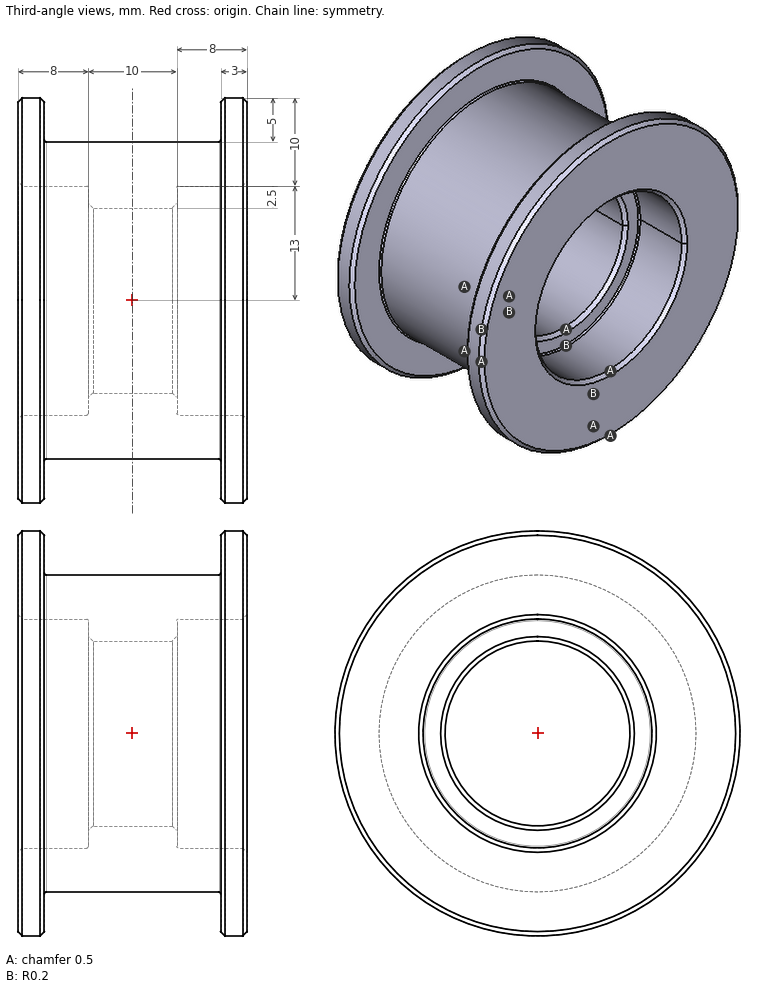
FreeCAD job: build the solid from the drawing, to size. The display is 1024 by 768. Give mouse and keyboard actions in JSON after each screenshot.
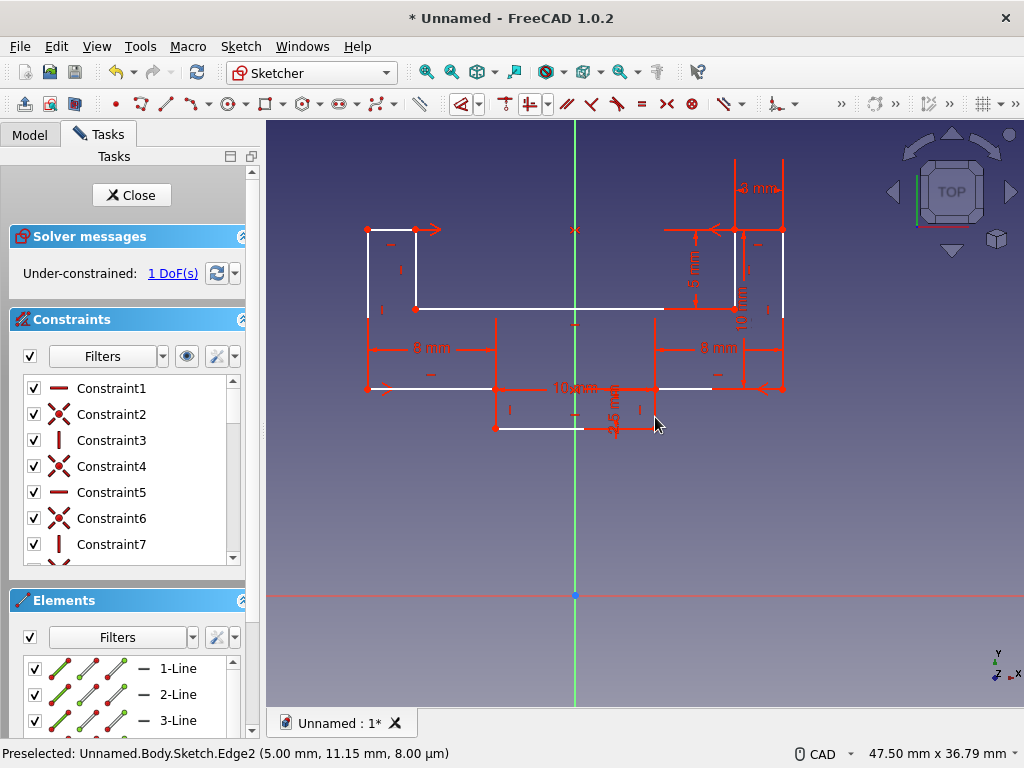
{"action": "left_click", "coordinate": [655, 389]}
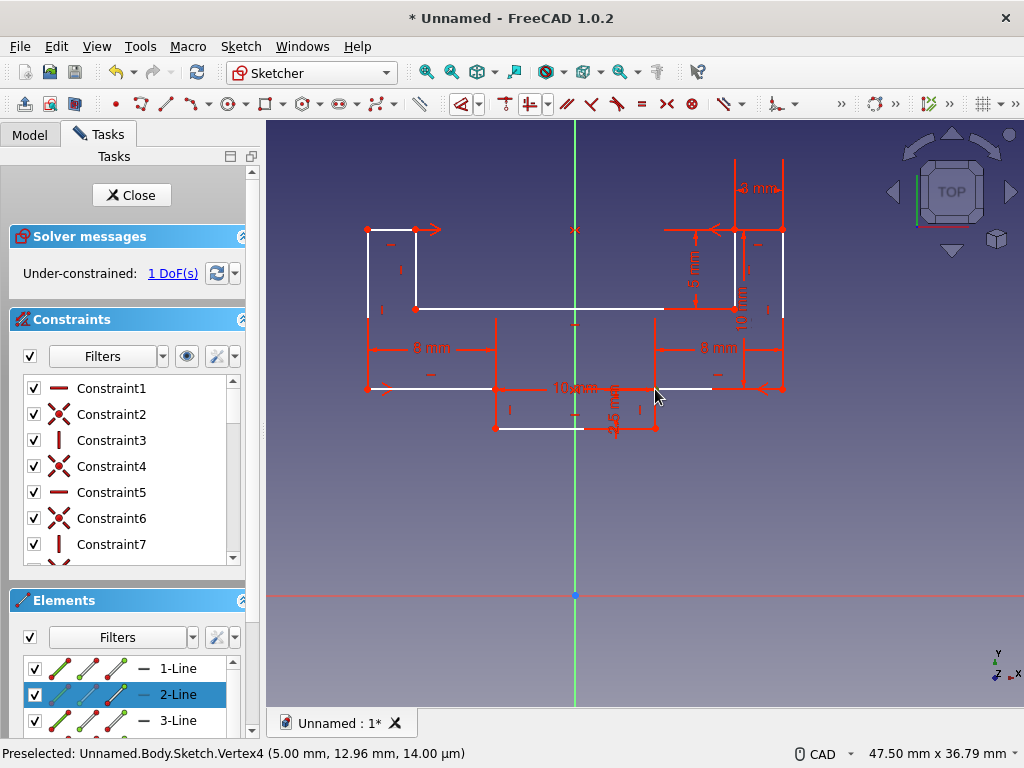
{"action": "key", "text": "i"}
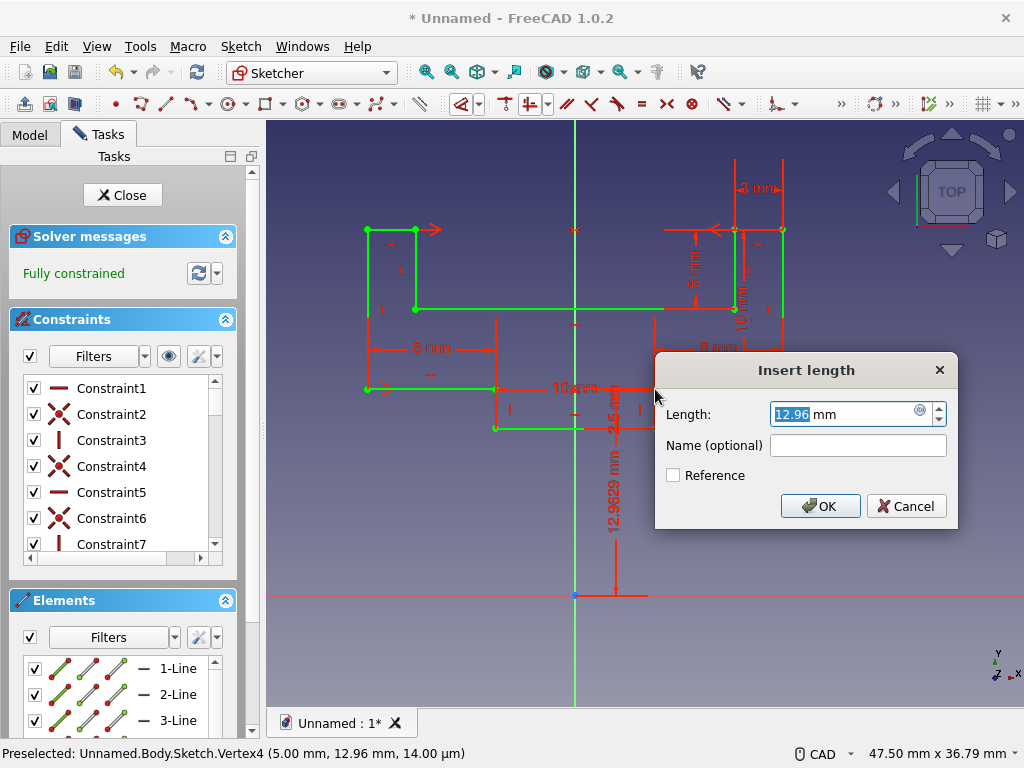
{"action": "type", "text": "13"}
{"action": "key", "text": "Return"}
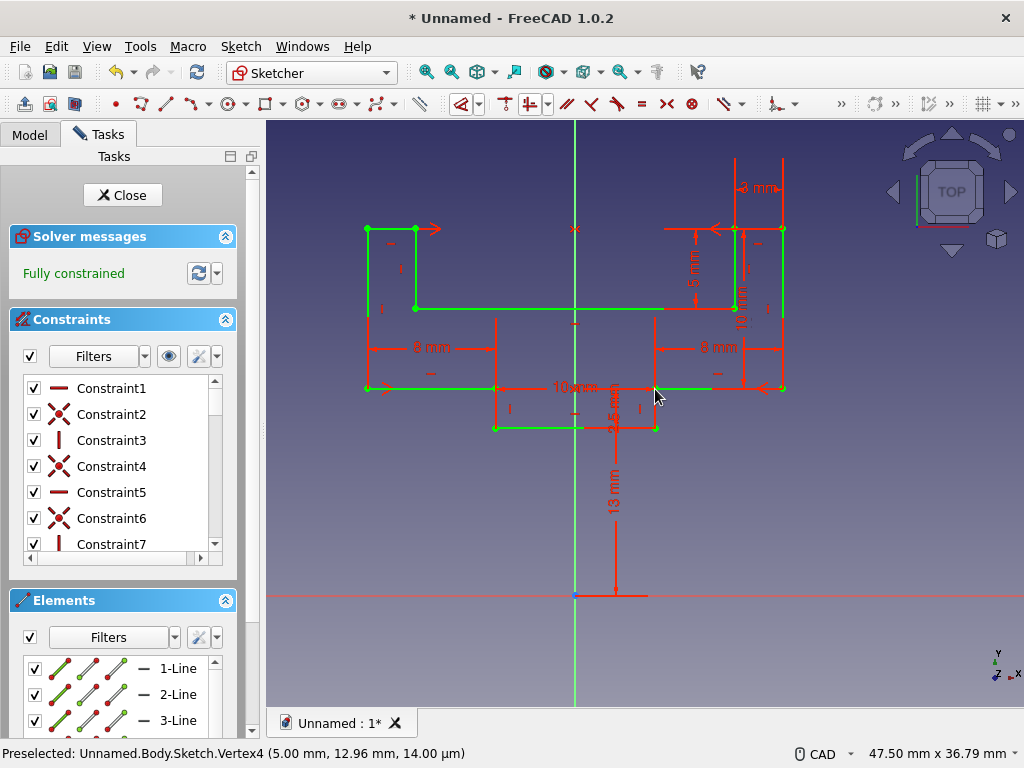
{"action": "left_click", "coordinate": [123, 195]}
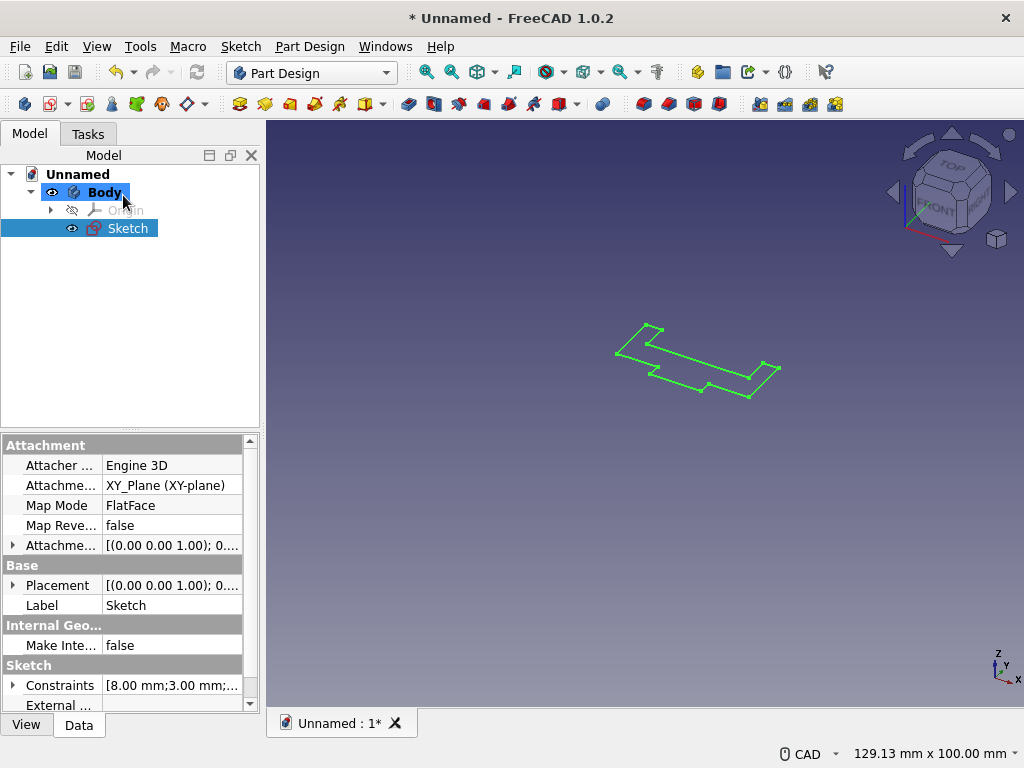
{"action": "left_click", "coordinate": [265, 104]}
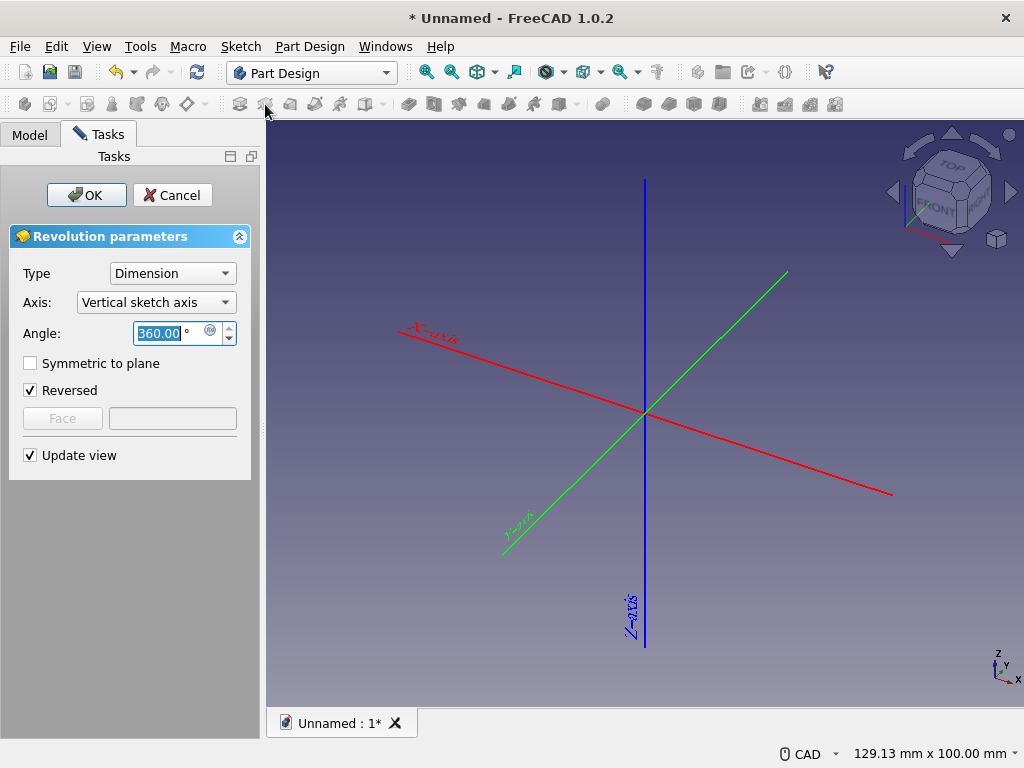
{"action": "left_click", "coordinate": [157, 302]}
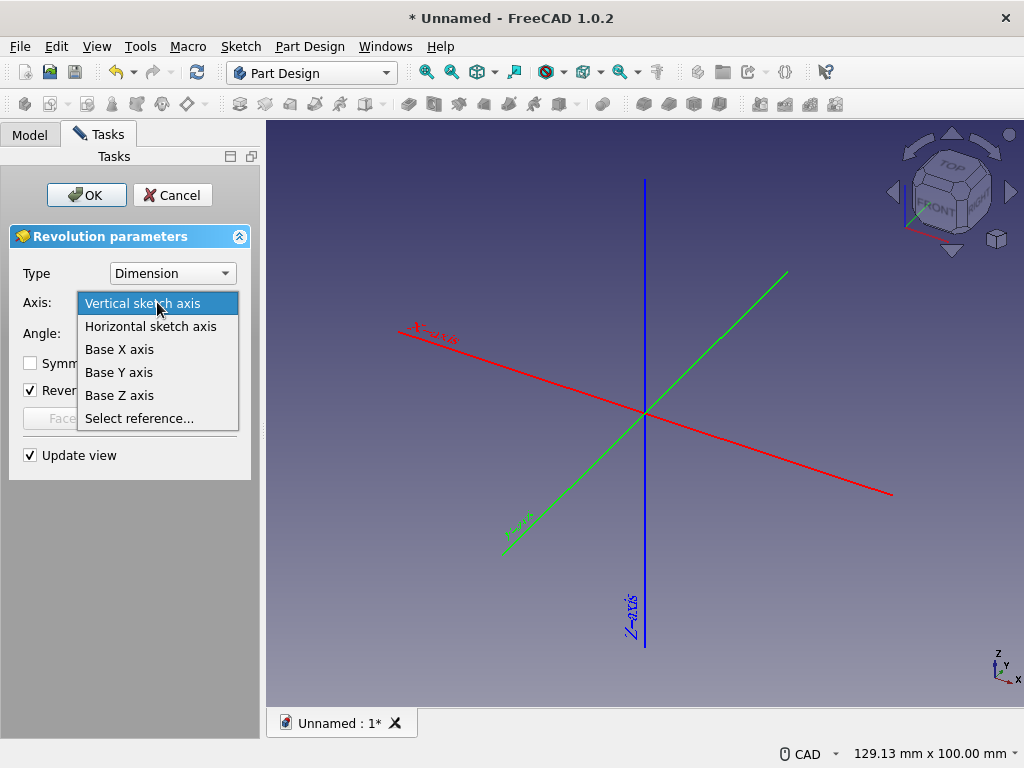
{"action": "left_click", "coordinate": [156, 326]}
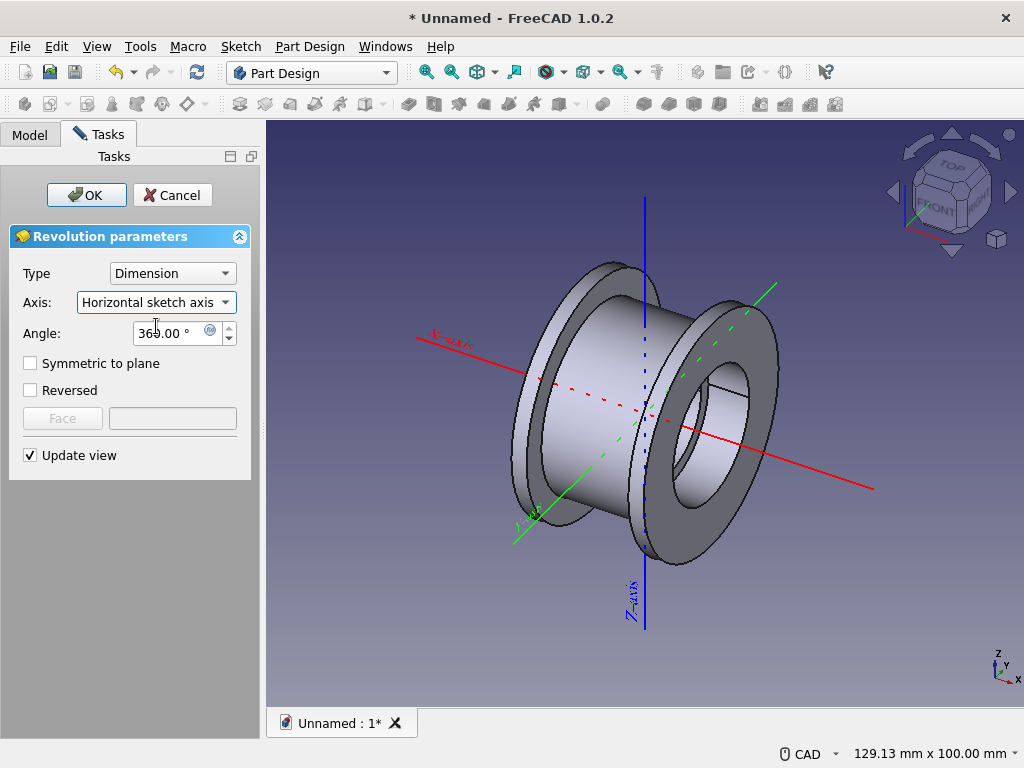
{"action": "left_click", "coordinate": [87, 195]}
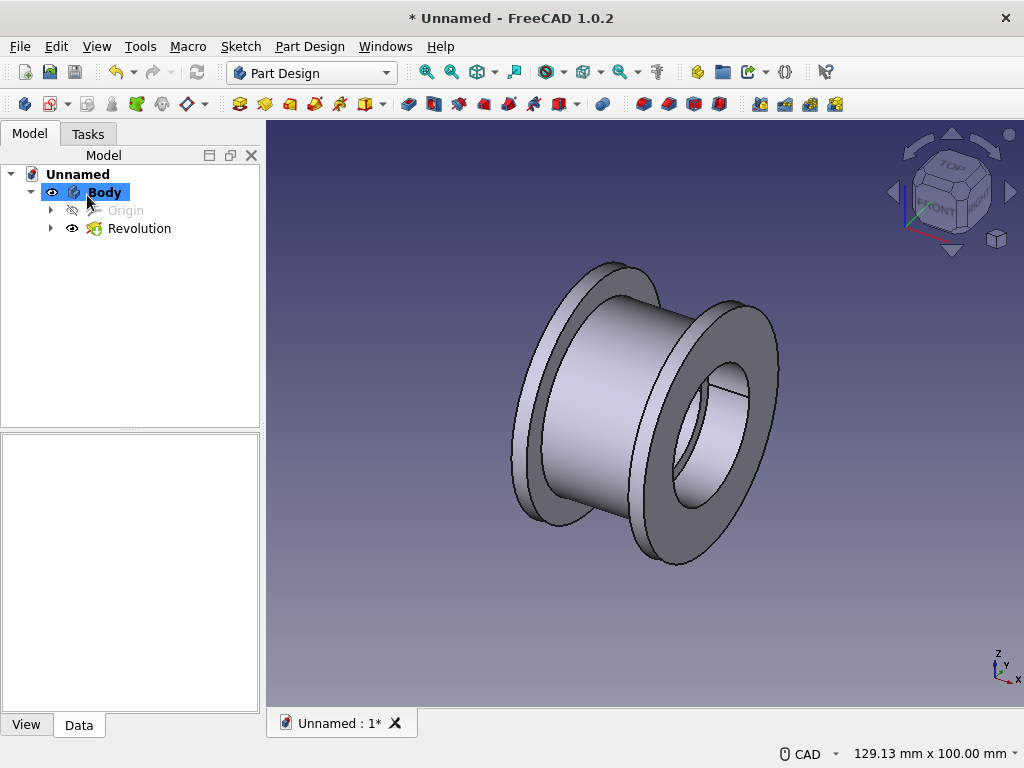
{"action": "left_click", "coordinate": [699, 506]}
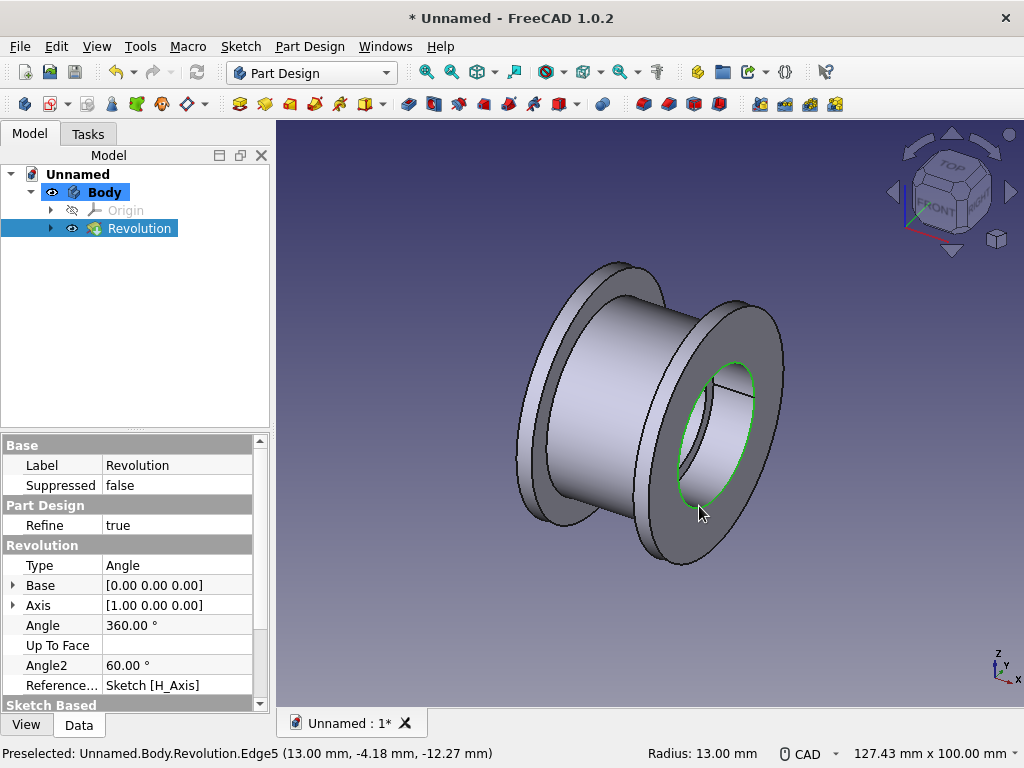
{"action": "left_click", "coordinate": [649, 501], "text": "ctrl"}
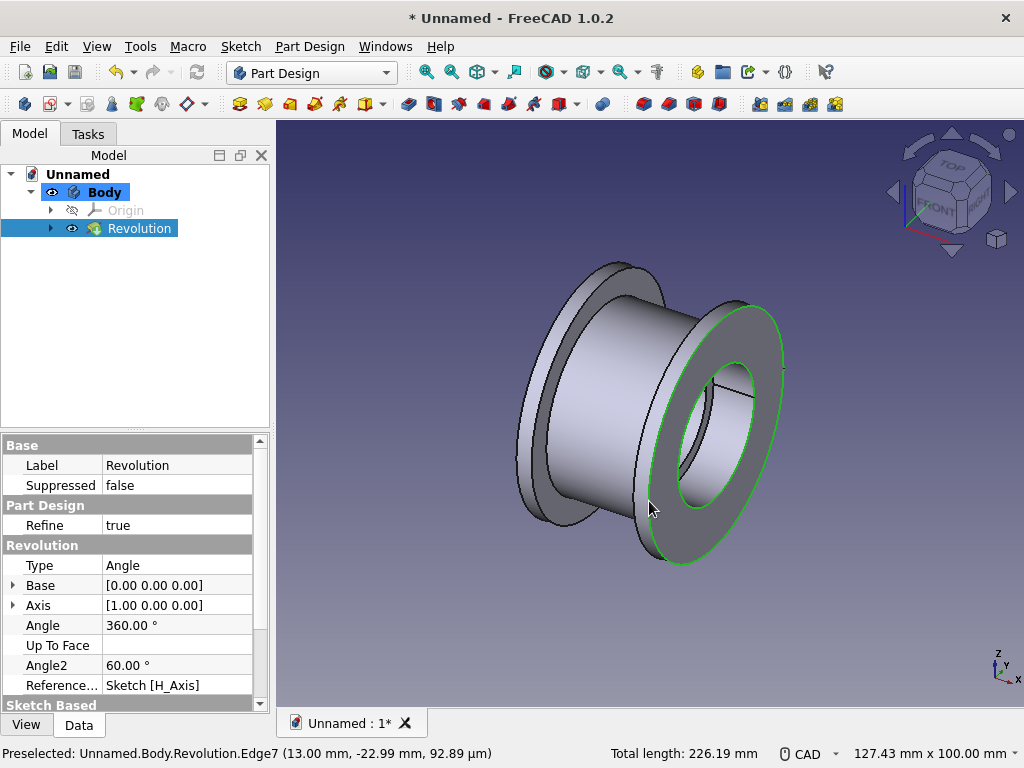
{"action": "left_click", "coordinate": [722, 303], "text": "ctrl"}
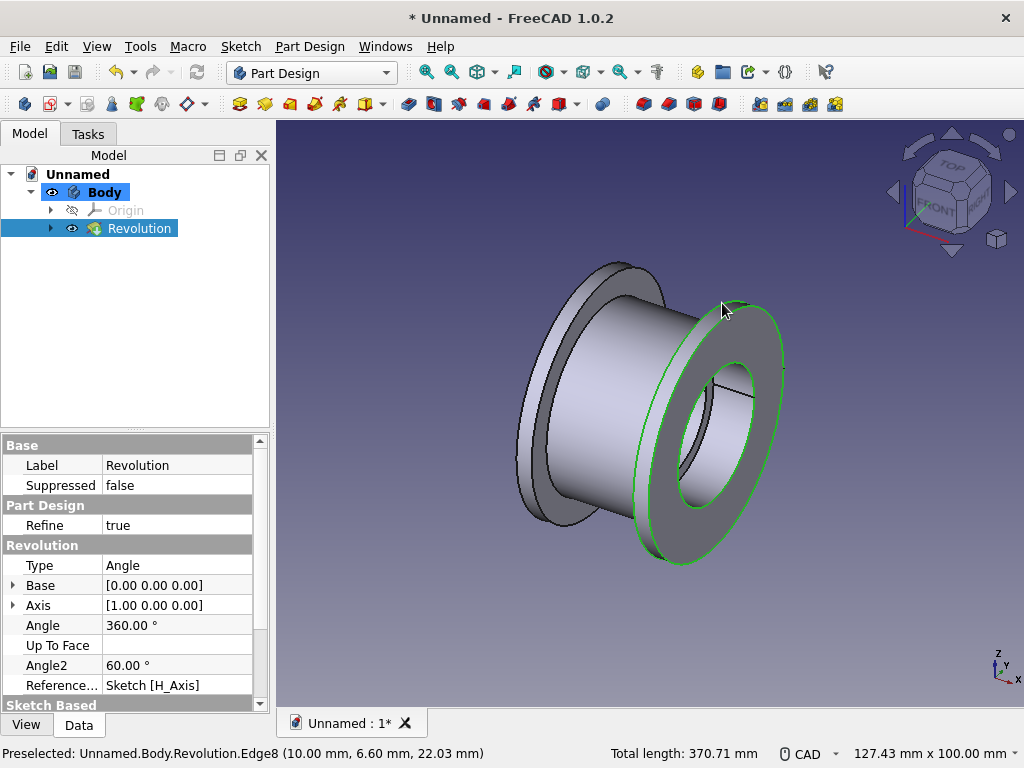
{"action": "left_click", "coordinate": [532, 463], "text": "ctrl"}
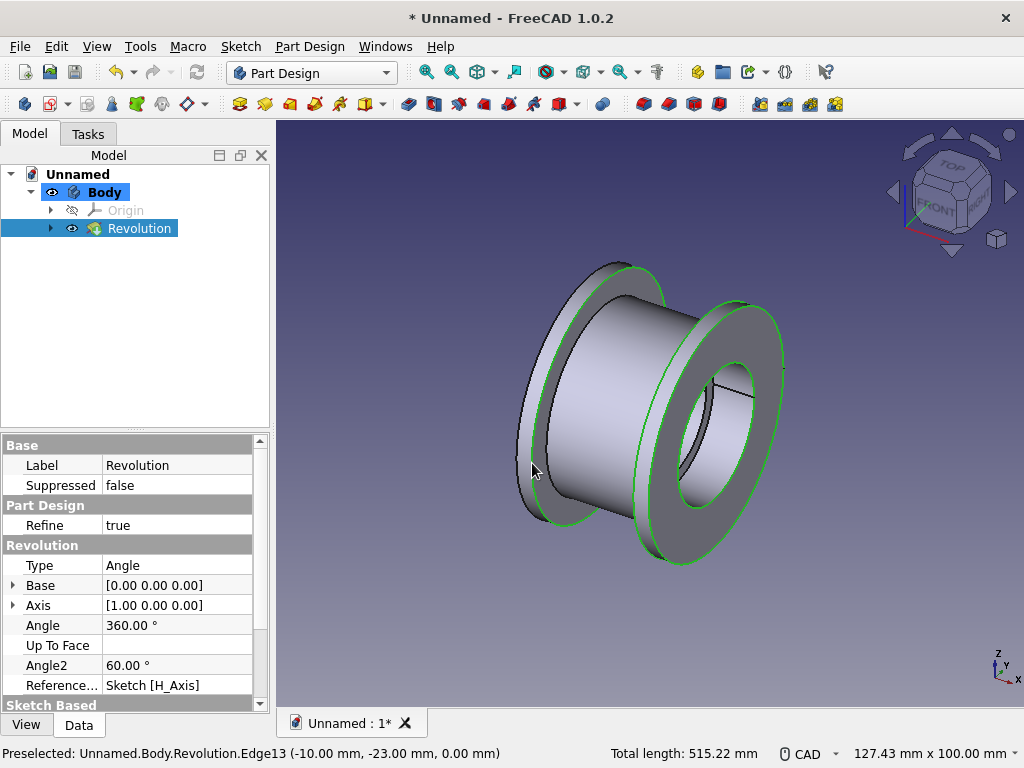
{"action": "left_click", "coordinate": [685, 459], "text": "ctrl"}